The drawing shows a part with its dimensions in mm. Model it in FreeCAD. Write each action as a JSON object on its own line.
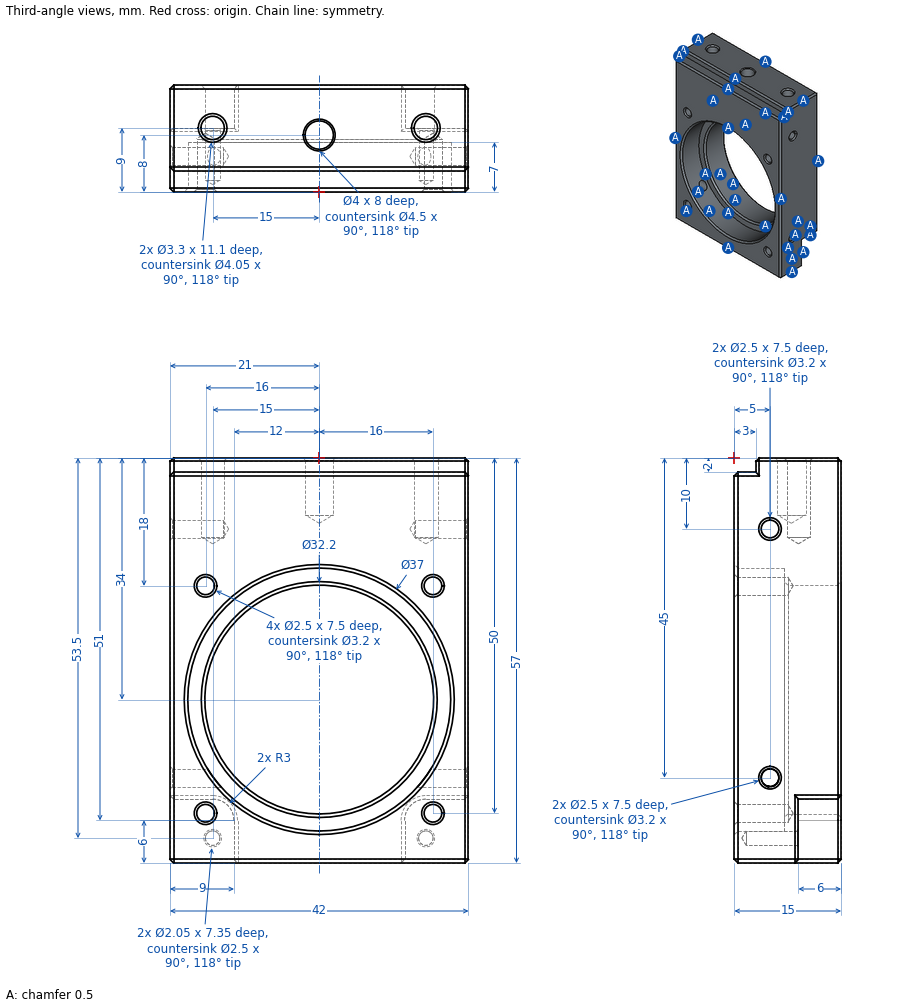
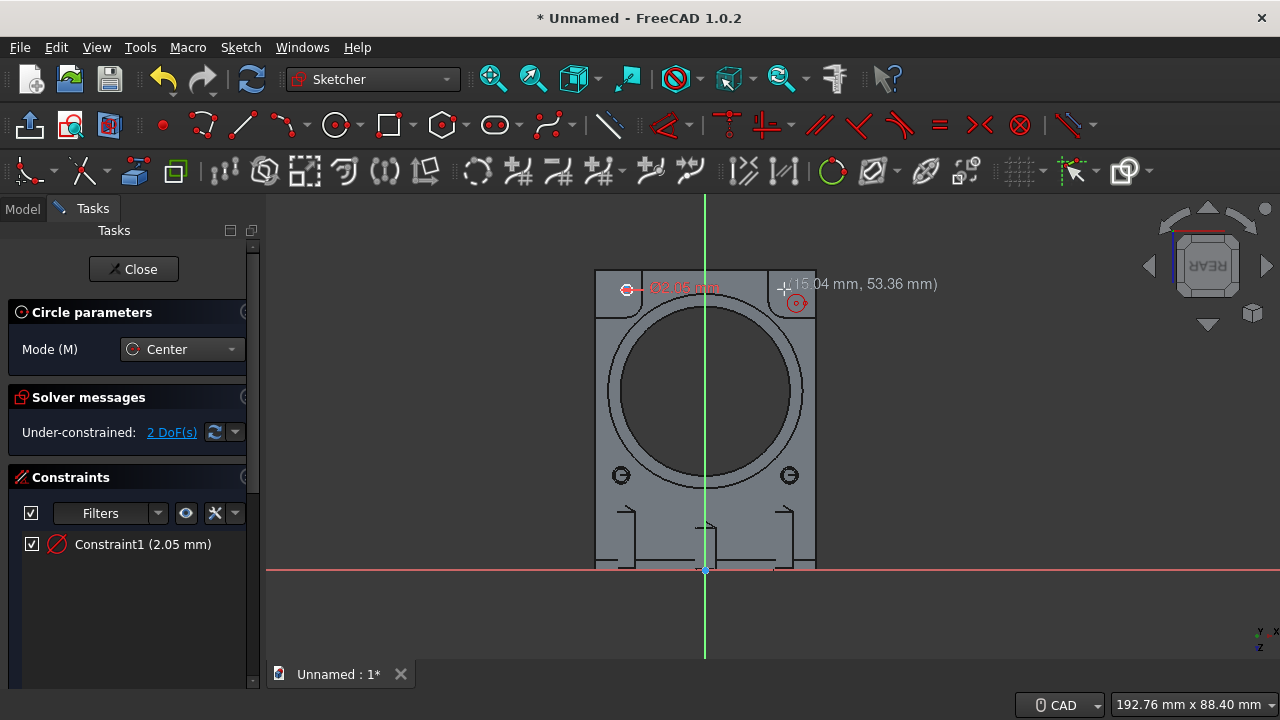
{"action": "left_click", "coordinate": [784, 289]}
{"action": "mouse_move", "coordinate": [788, 285]}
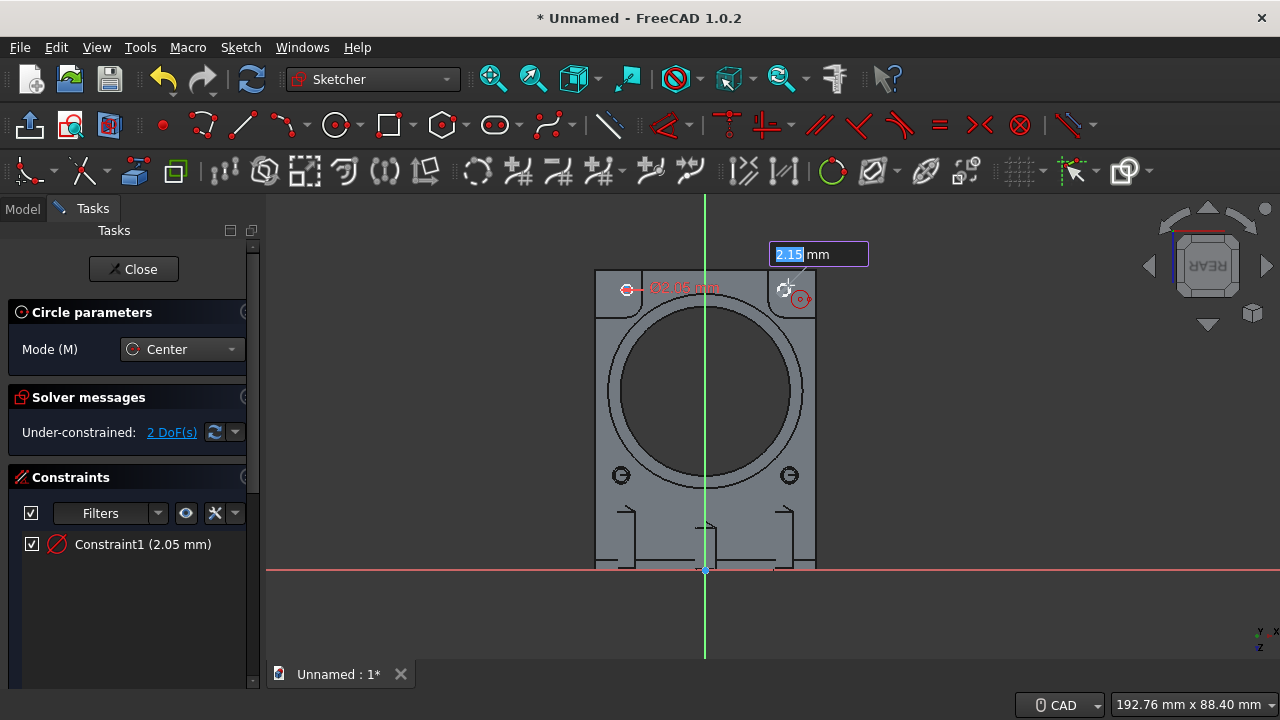
{"action": "type", "text": "2.05"}
{"action": "key", "text": "Return"}
{"action": "key", "text": "Escape"}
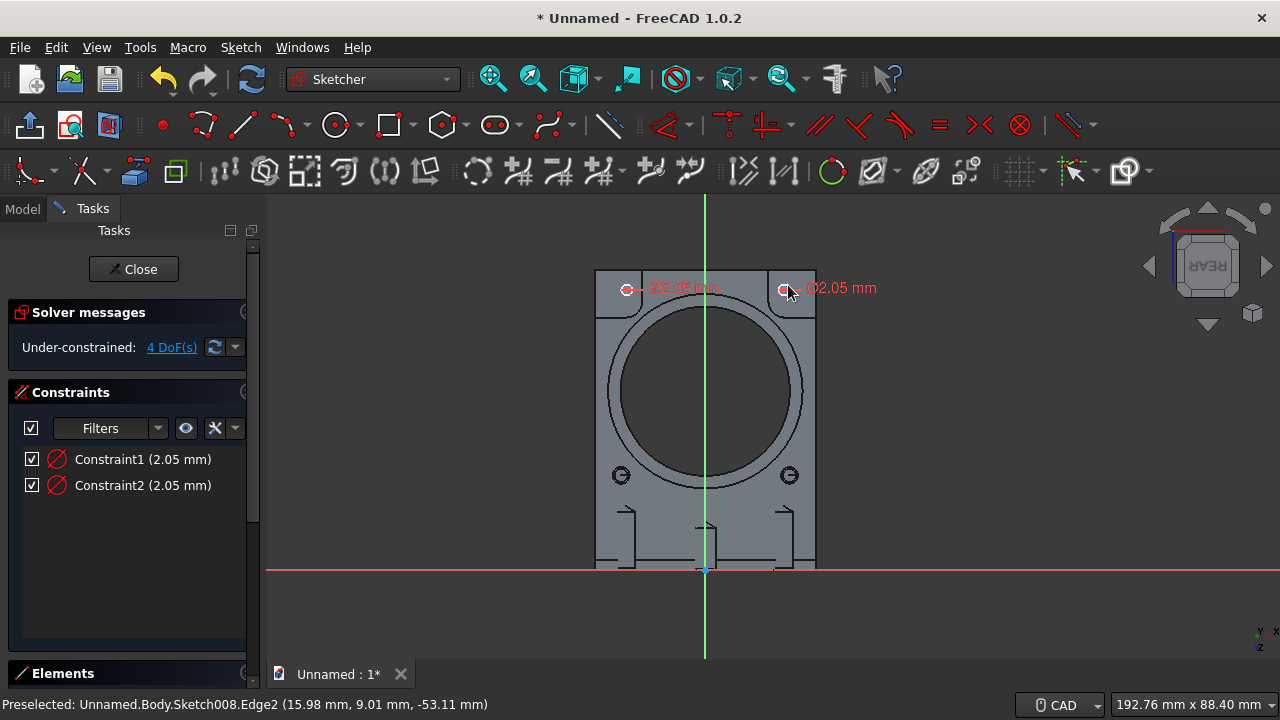
{"action": "left_click", "coordinate": [627, 290]}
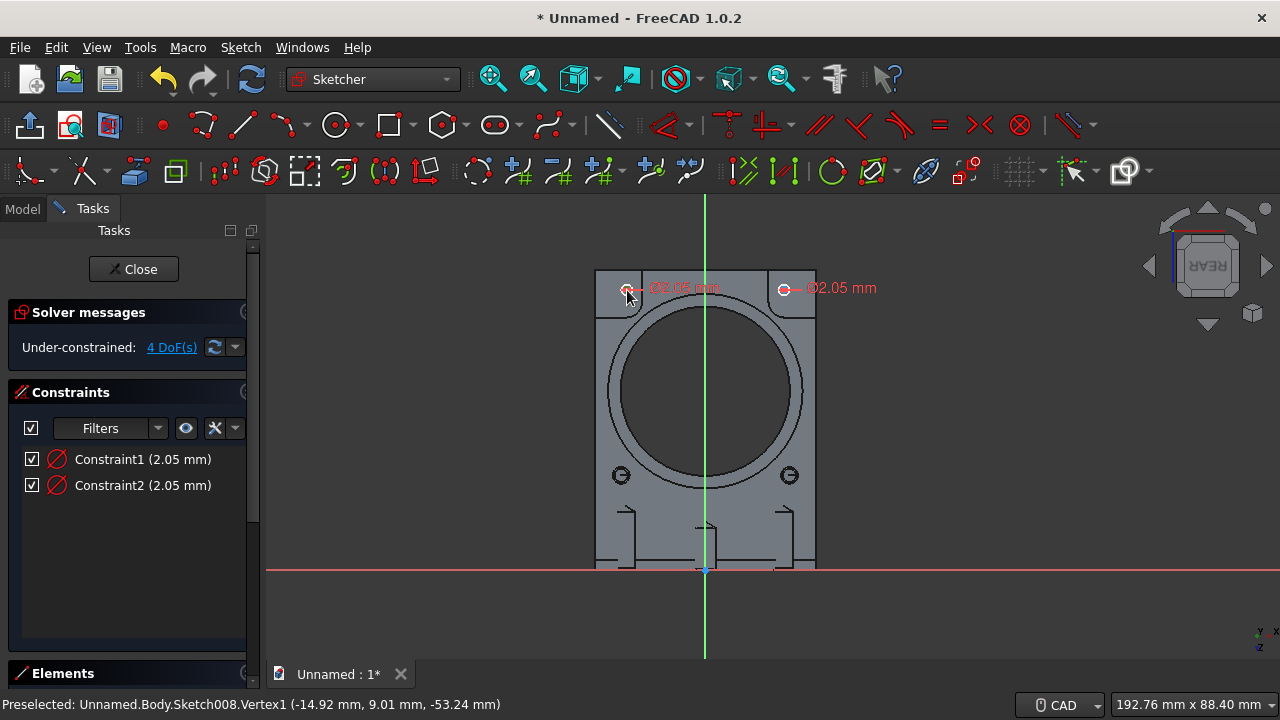
{"action": "left_click", "coordinate": [784, 290]}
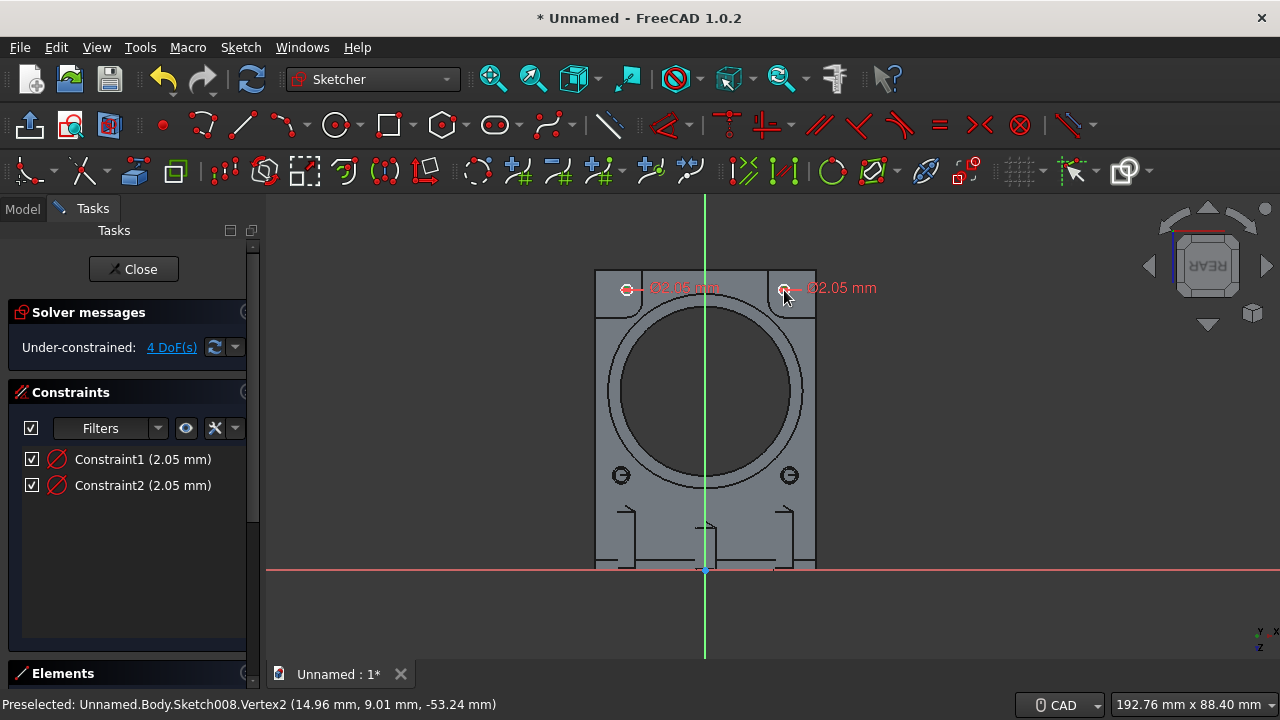
{"action": "left_click", "coordinate": [705, 602]}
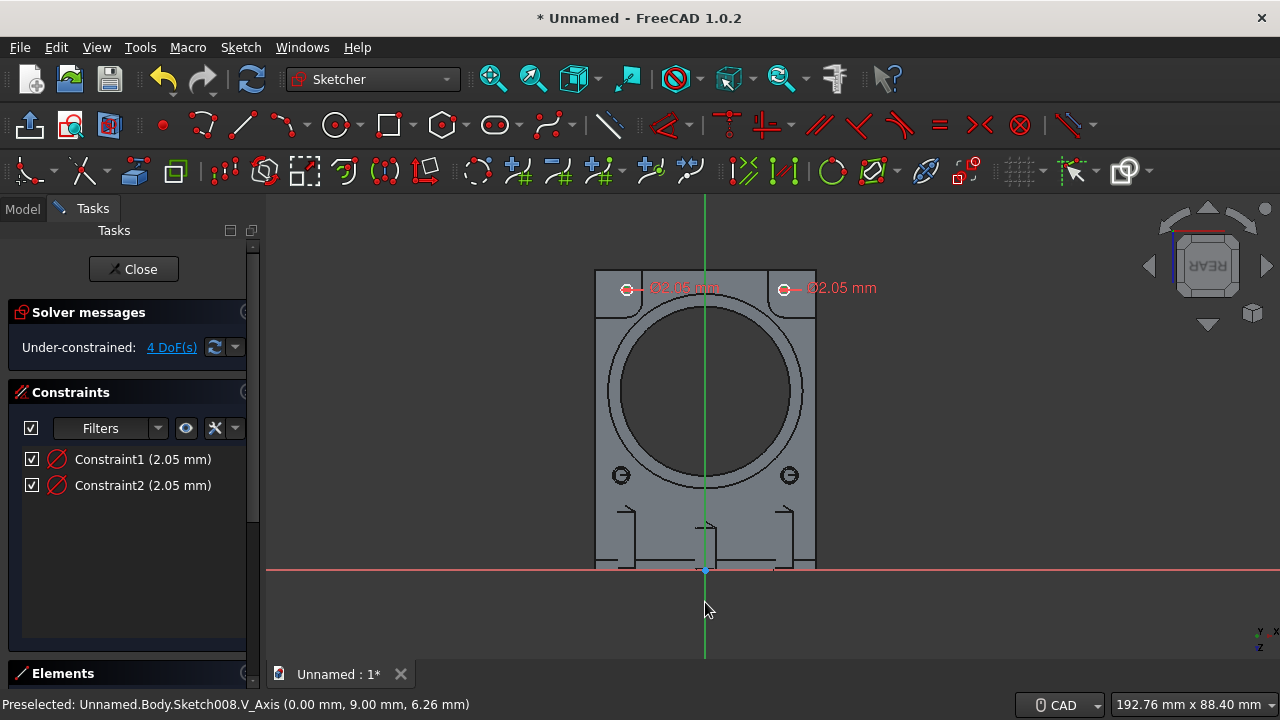
{"action": "left_click", "coordinate": [980, 126]}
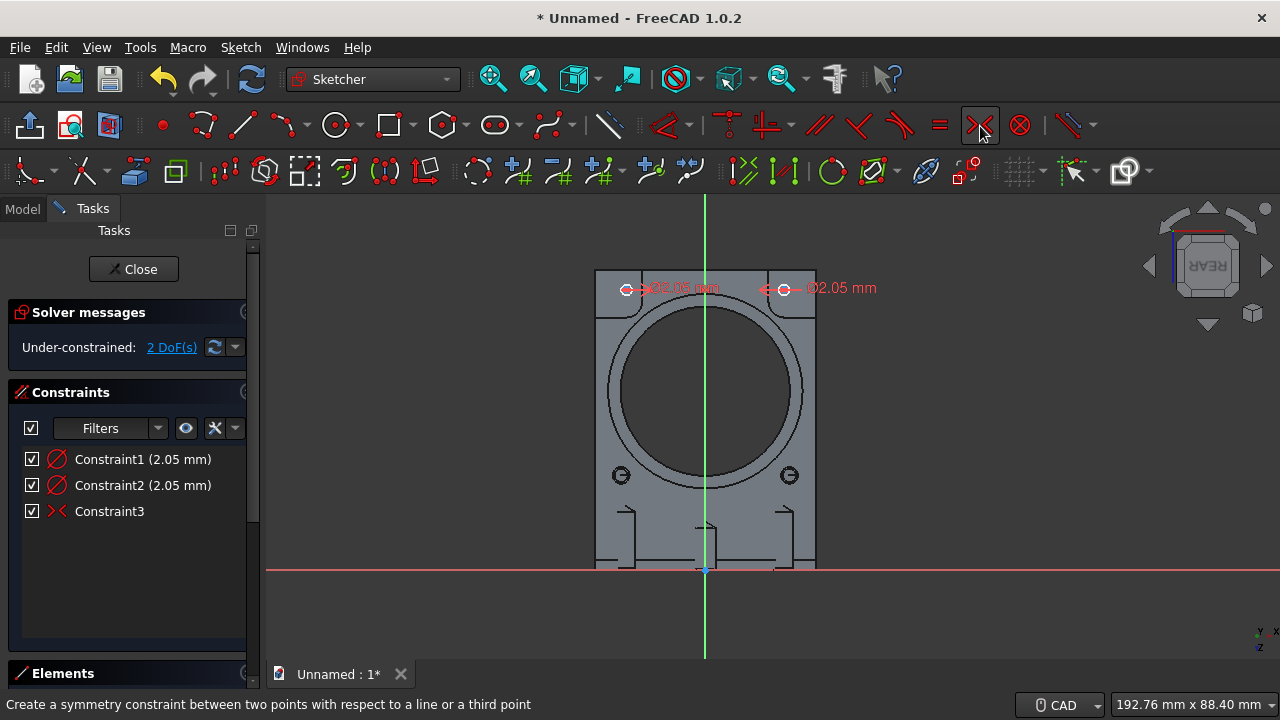
{"action": "key", "text": "d"}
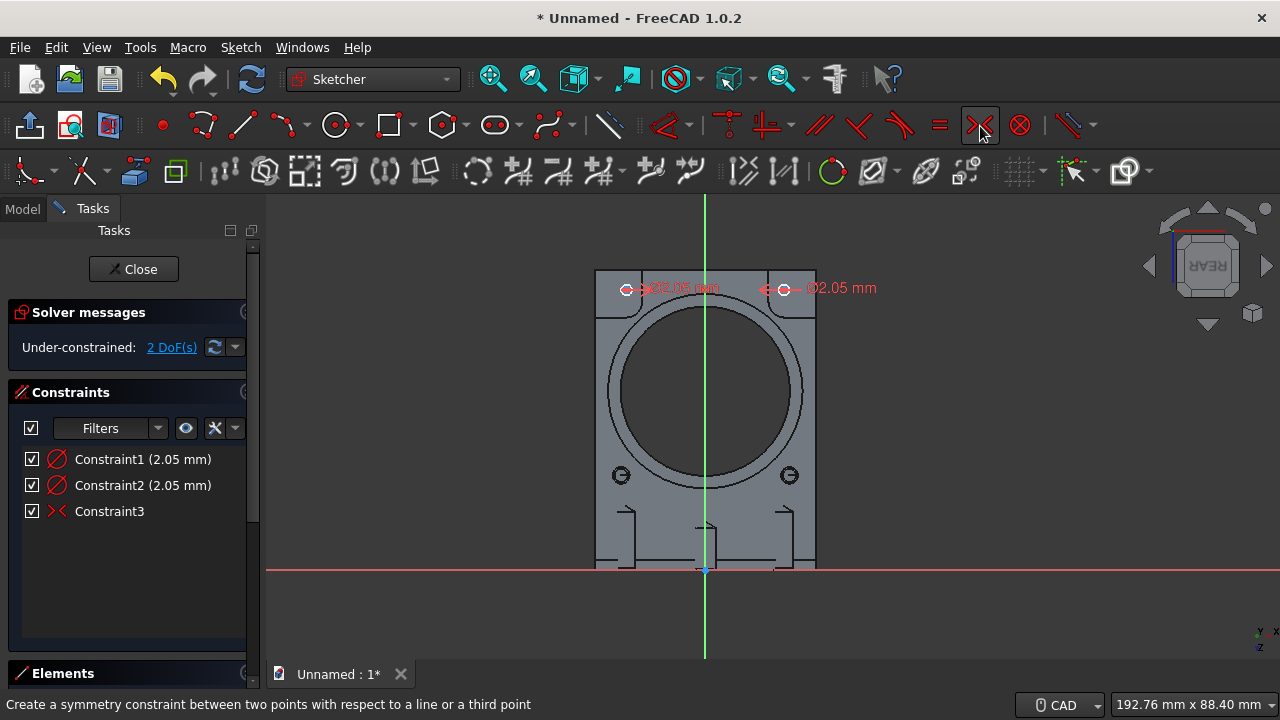
{"action": "left_click", "coordinate": [627, 290]}
{"action": "left_click", "coordinate": [666, 604]}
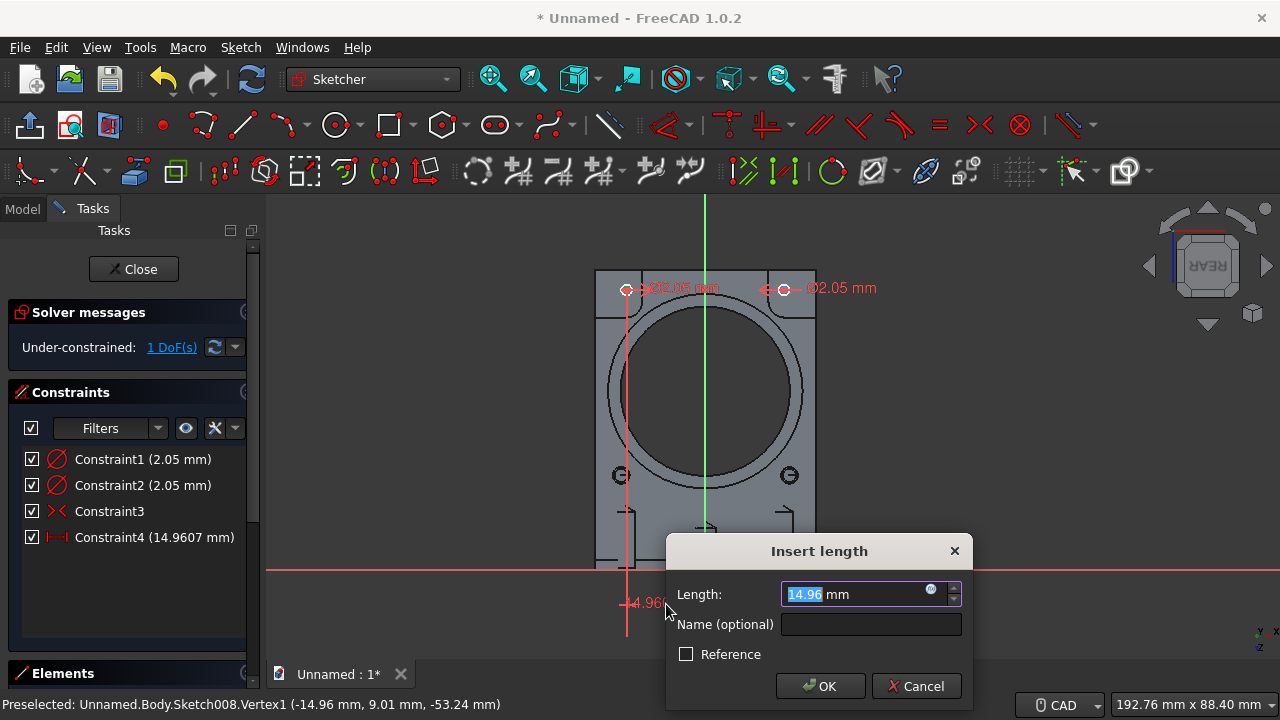
{"action": "type", "text": "15"}
{"action": "key", "text": "Return"}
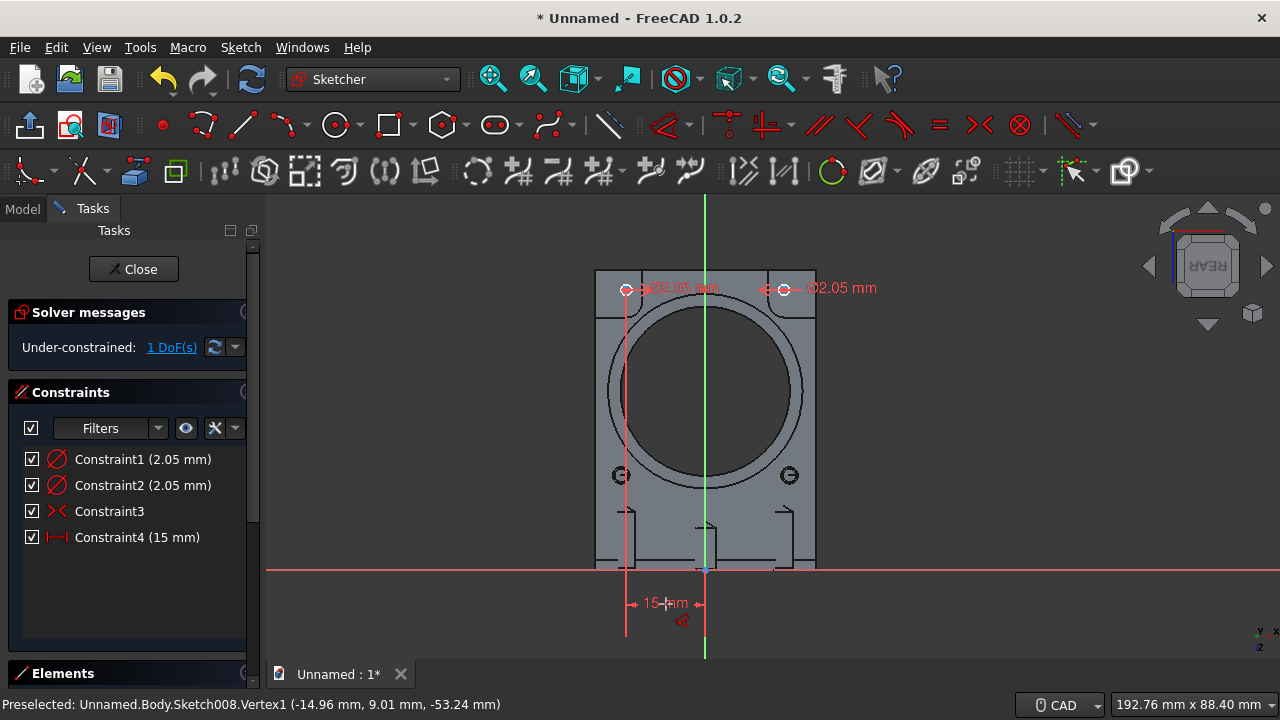
{"action": "left_click", "coordinate": [626, 290]}
{"action": "left_click", "coordinate": [592, 430]}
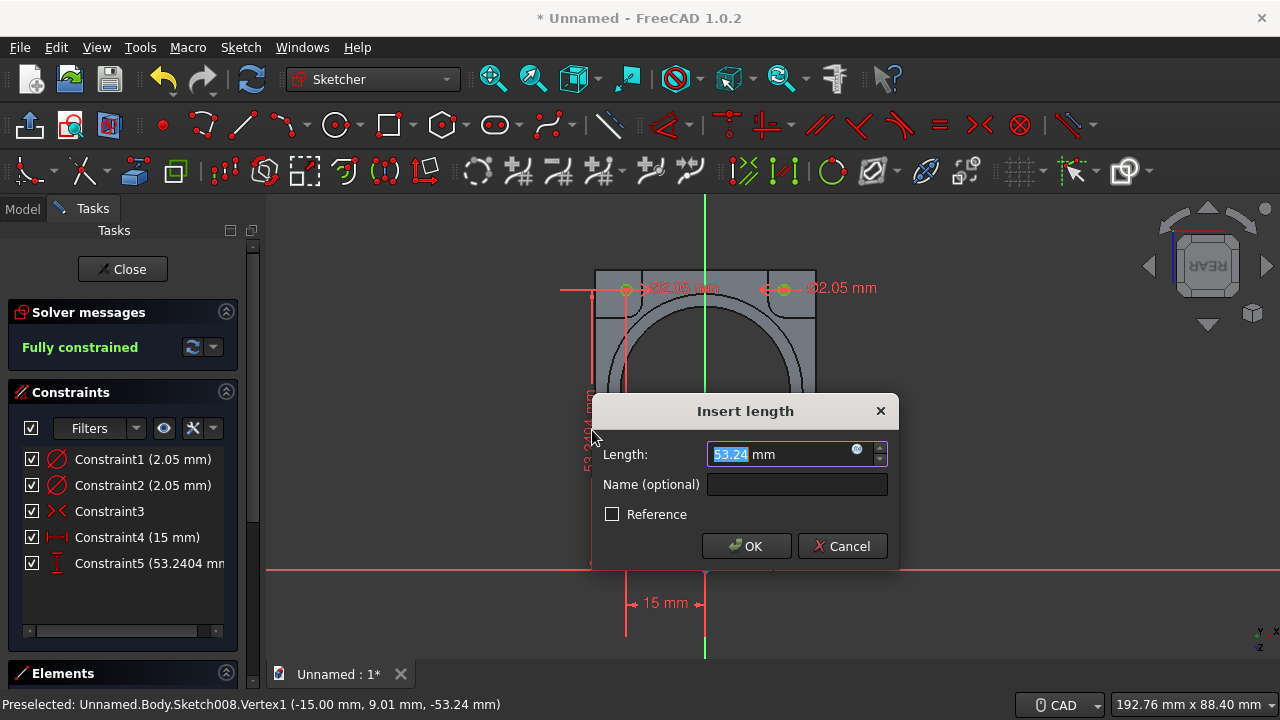
{"action": "type", "text": "53.5"}
{"action": "key", "text": "Return"}
{"action": "key", "text": "Escape"}